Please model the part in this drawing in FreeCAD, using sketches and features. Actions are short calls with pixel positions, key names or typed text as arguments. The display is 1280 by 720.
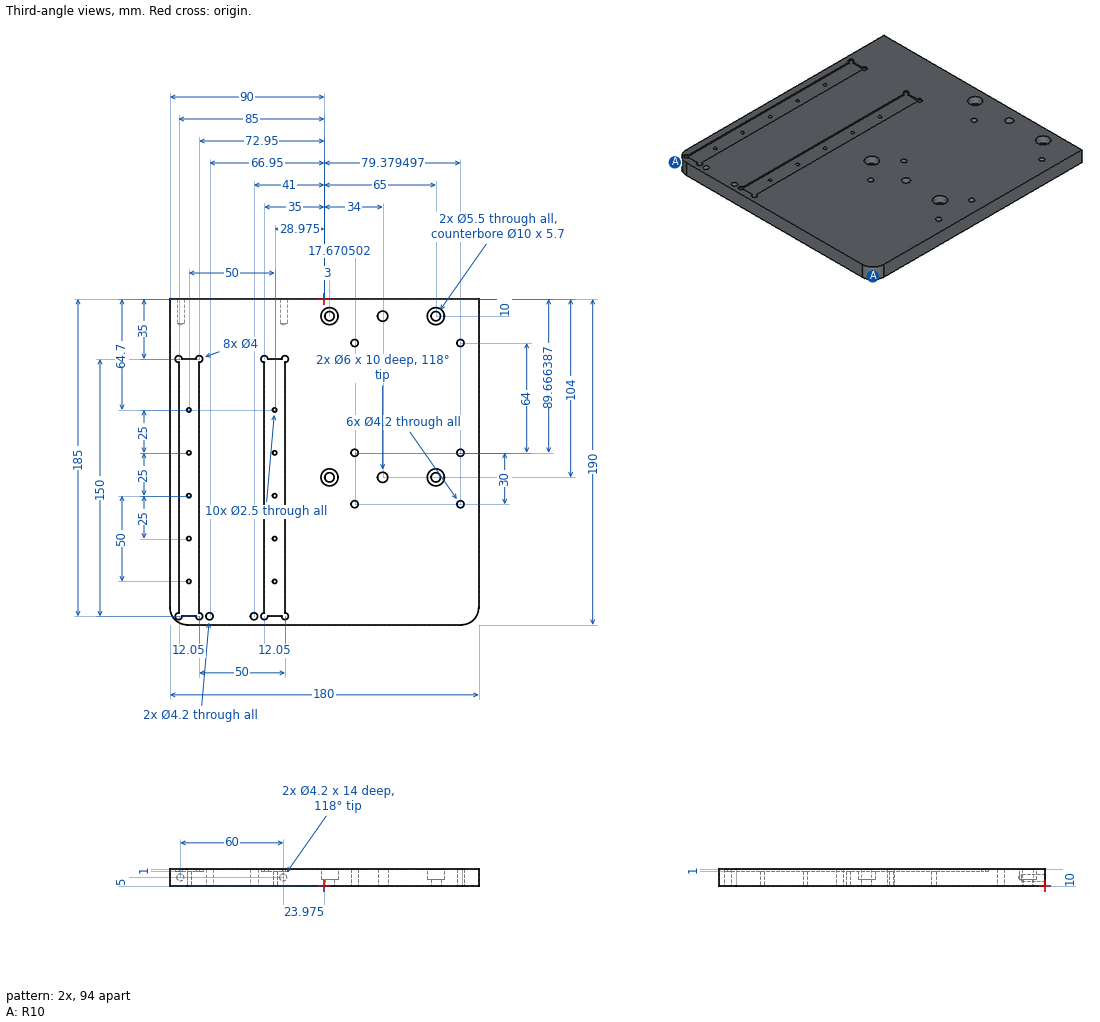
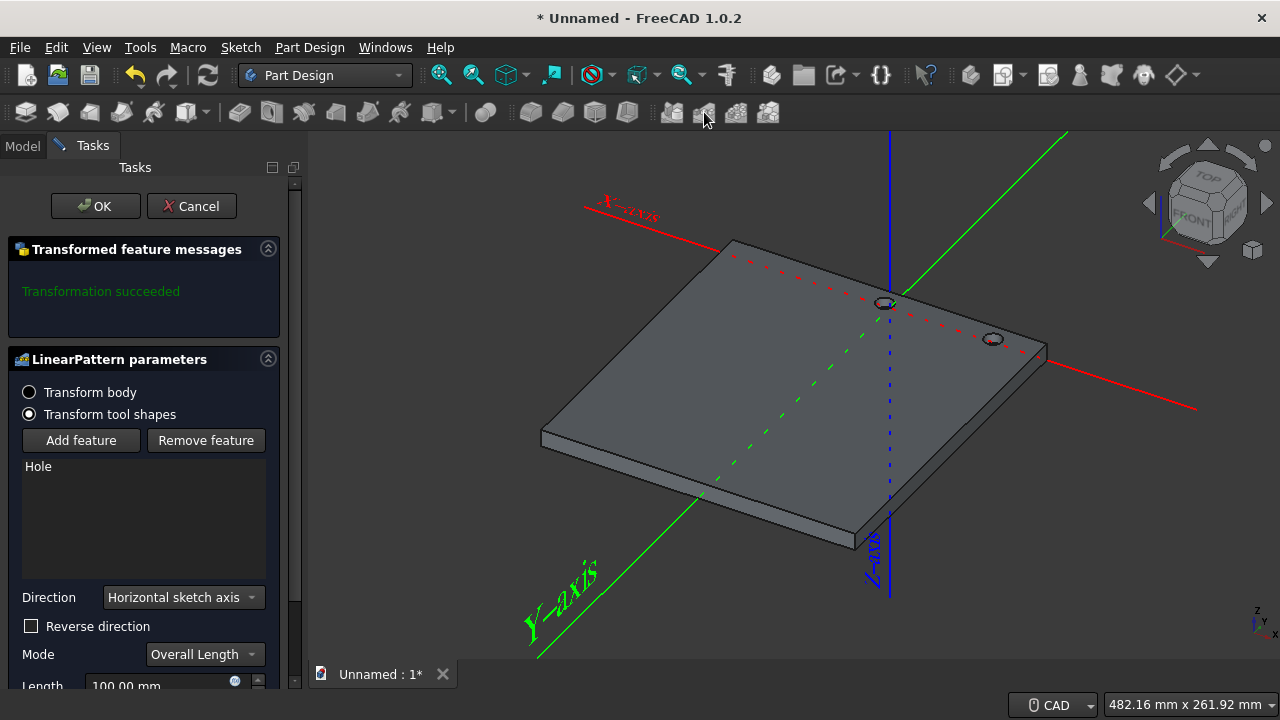
click(184, 598)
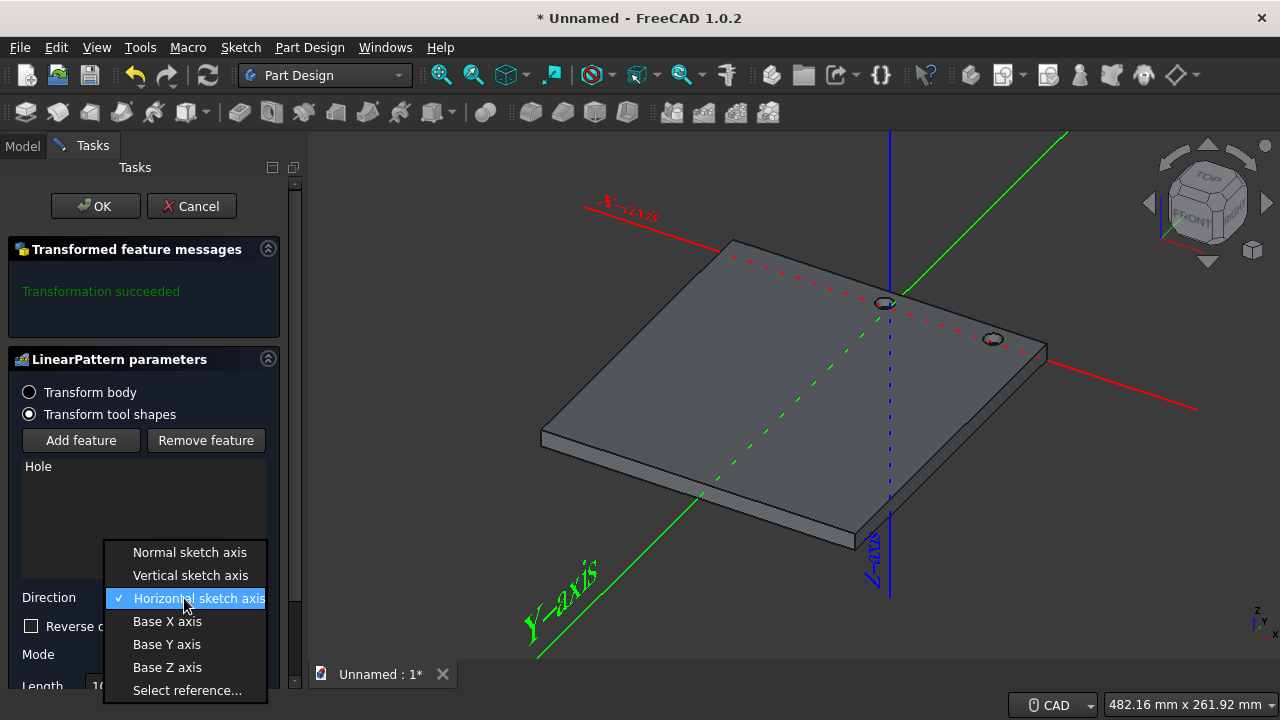
click(184, 644)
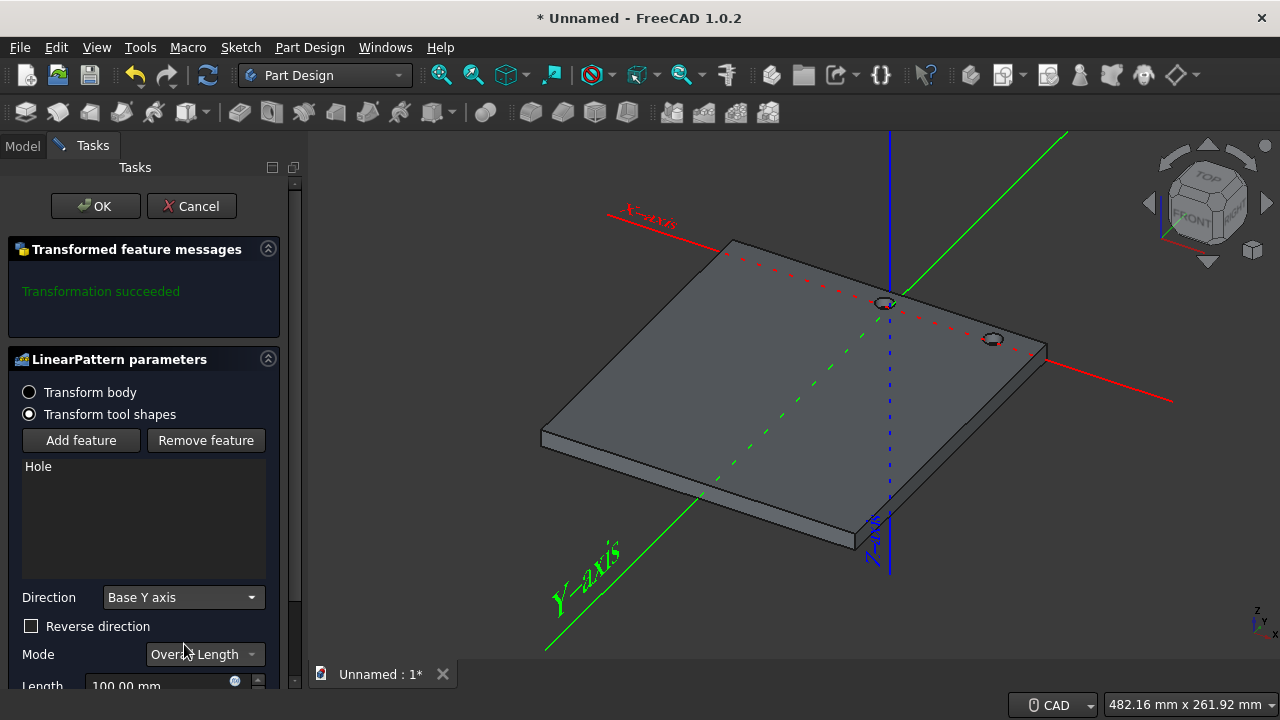
click(206, 654)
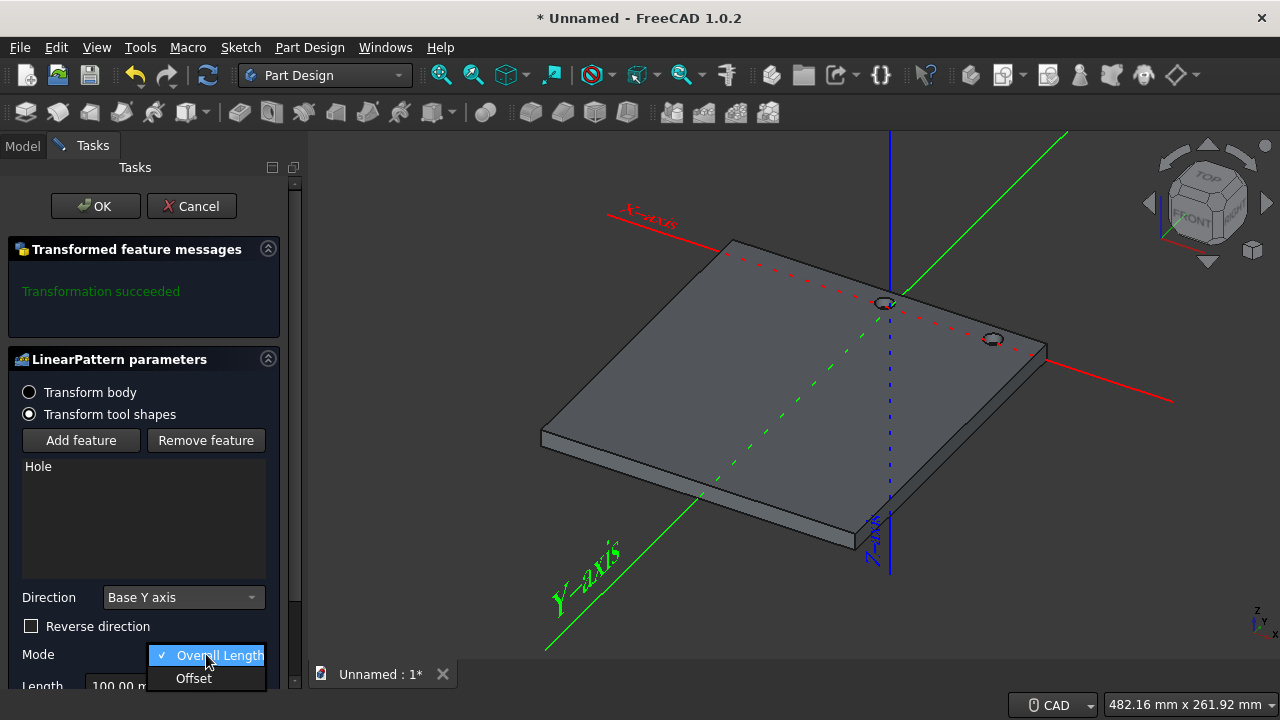
click(206, 678)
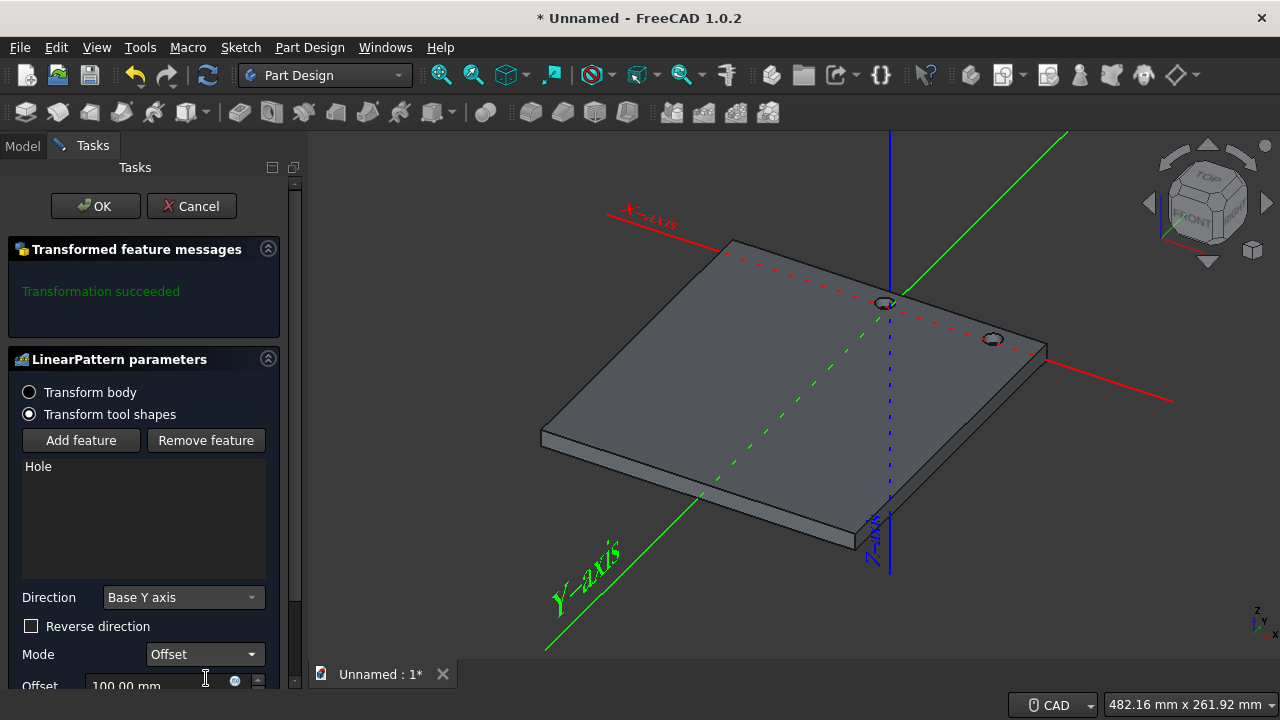
scroll(295, 432, down, 2)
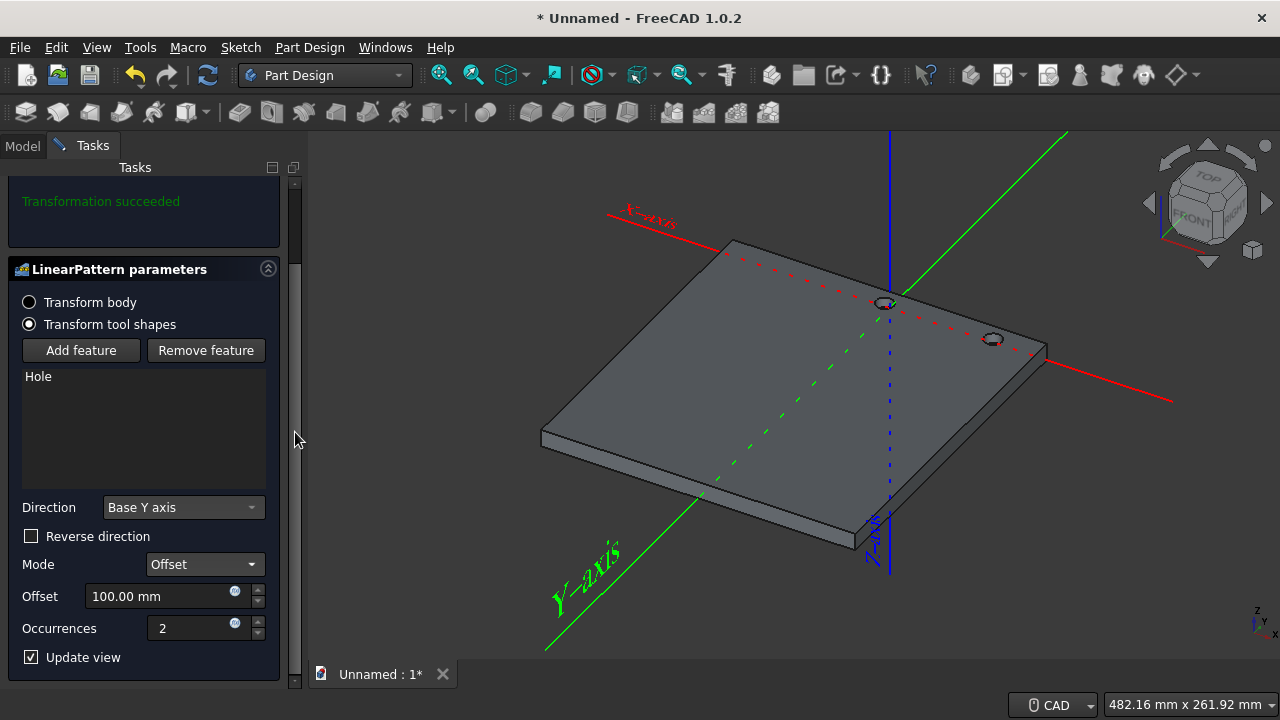
triple_click(168, 596)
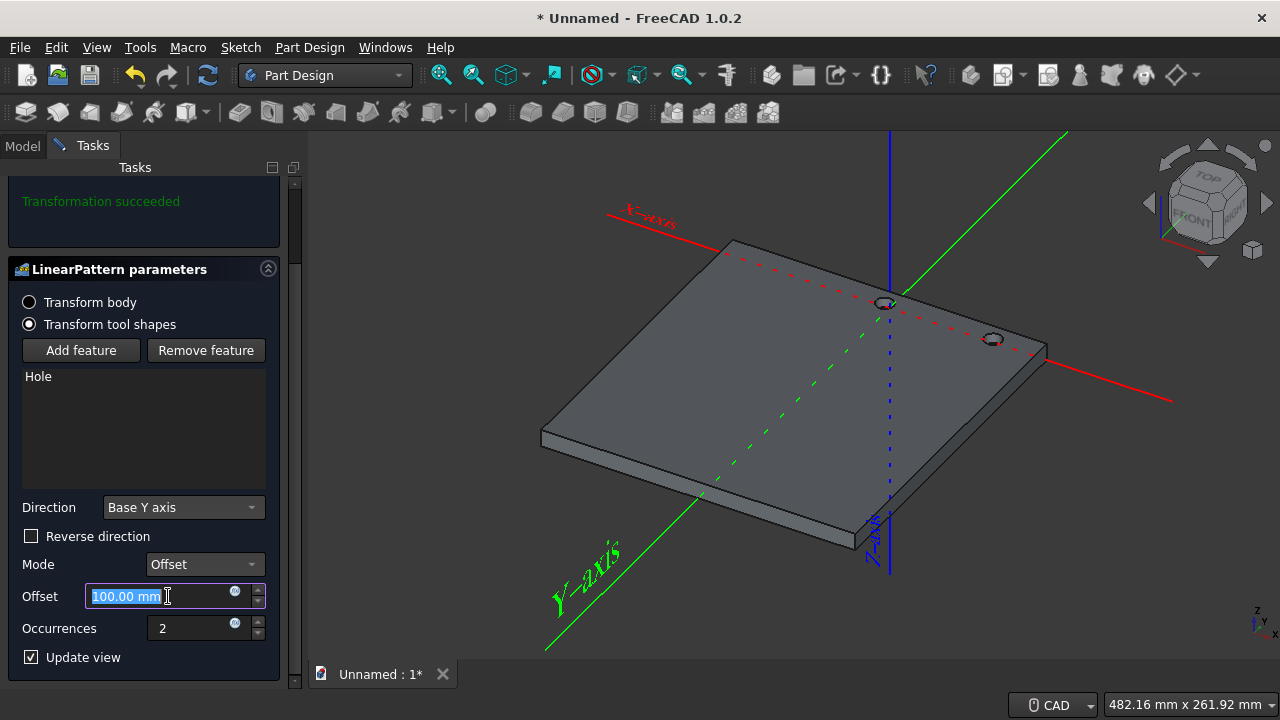
text(94)
key(Tab)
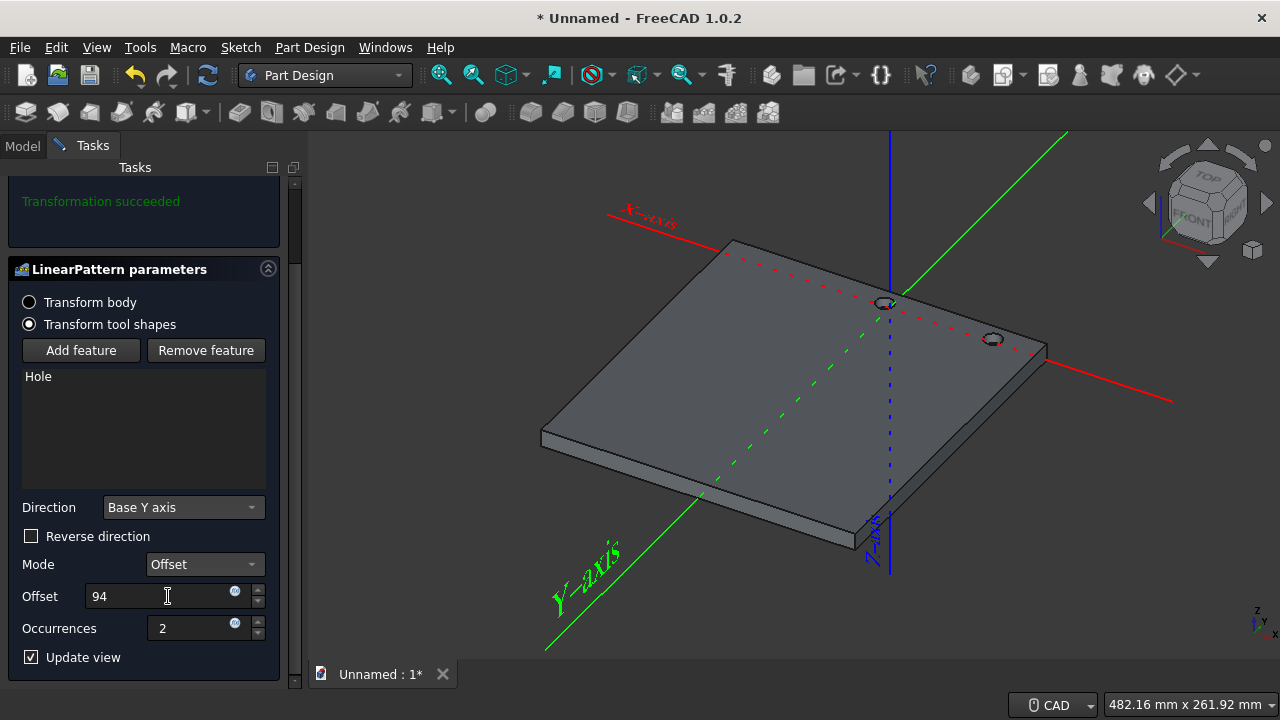
triple_click(198, 628)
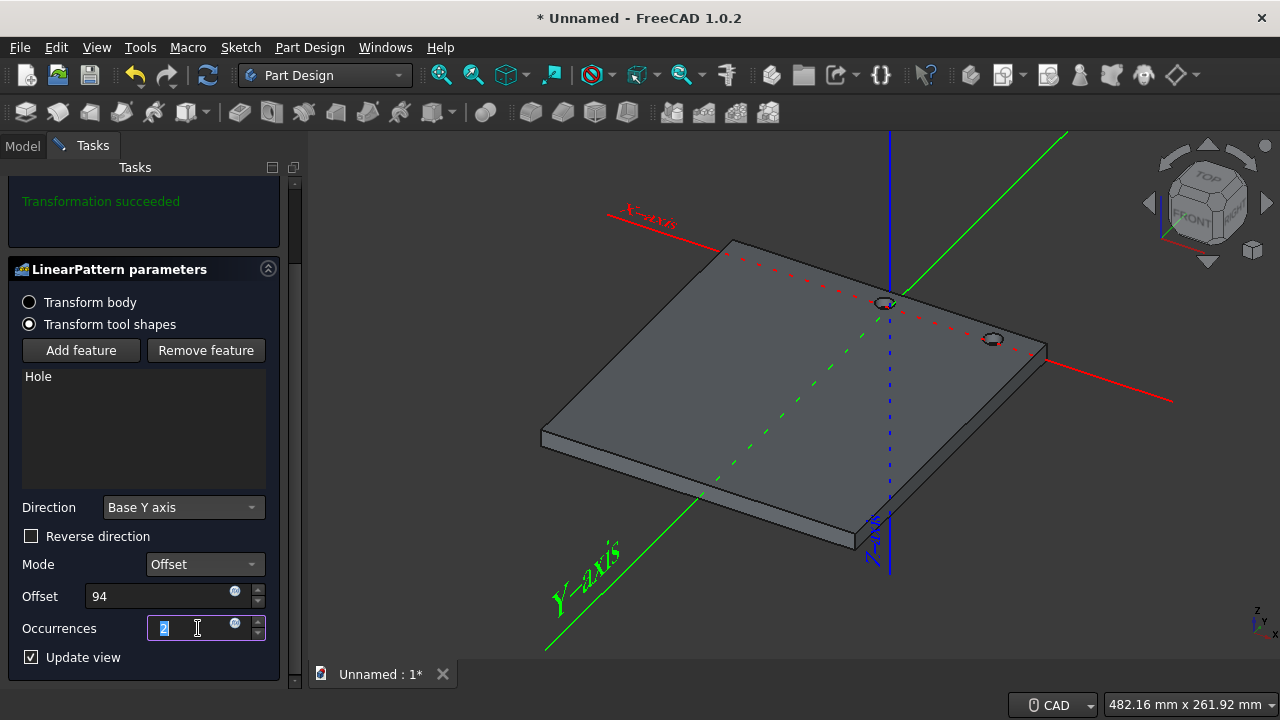
text(2)
key(Tab)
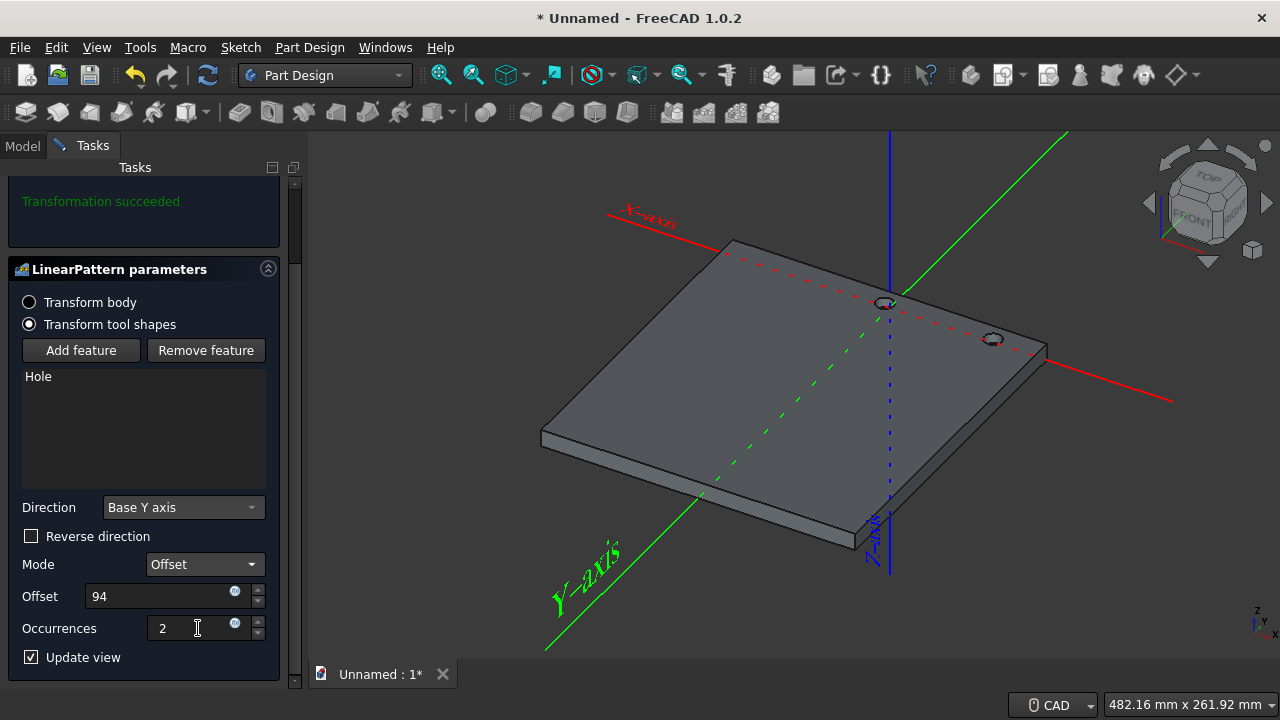
click(30, 536)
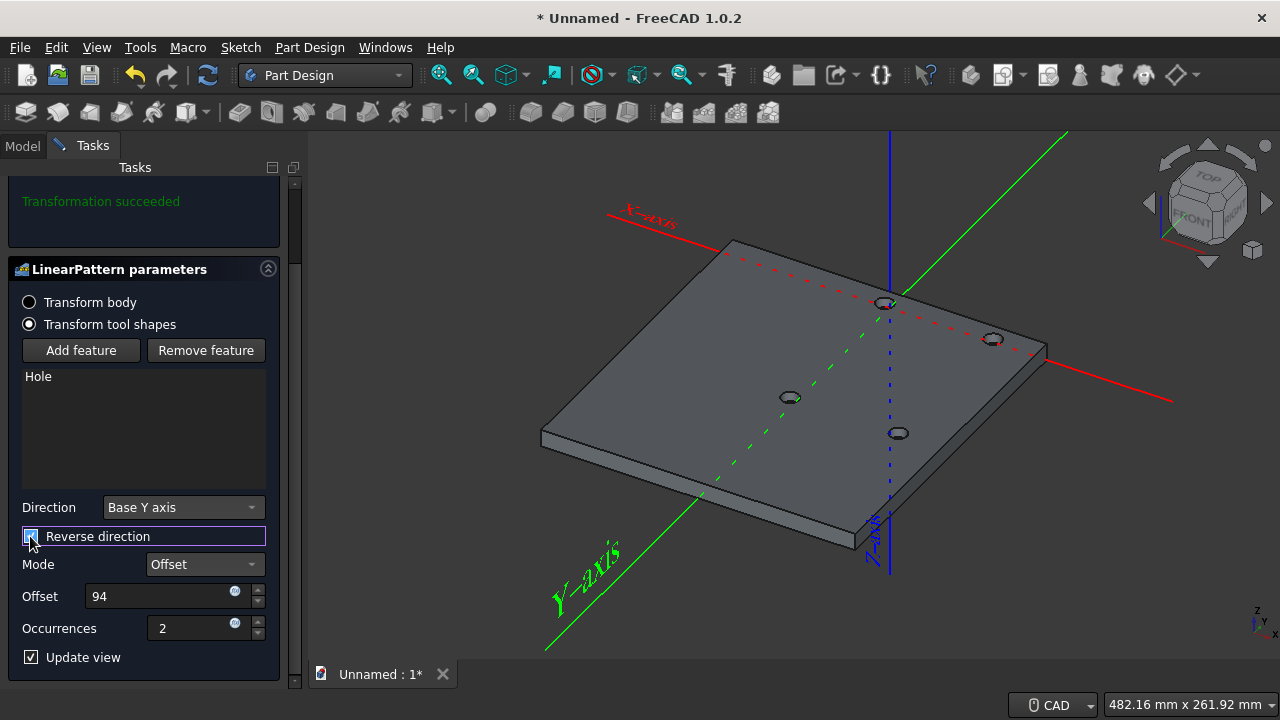
scroll(295, 432, up, 3)